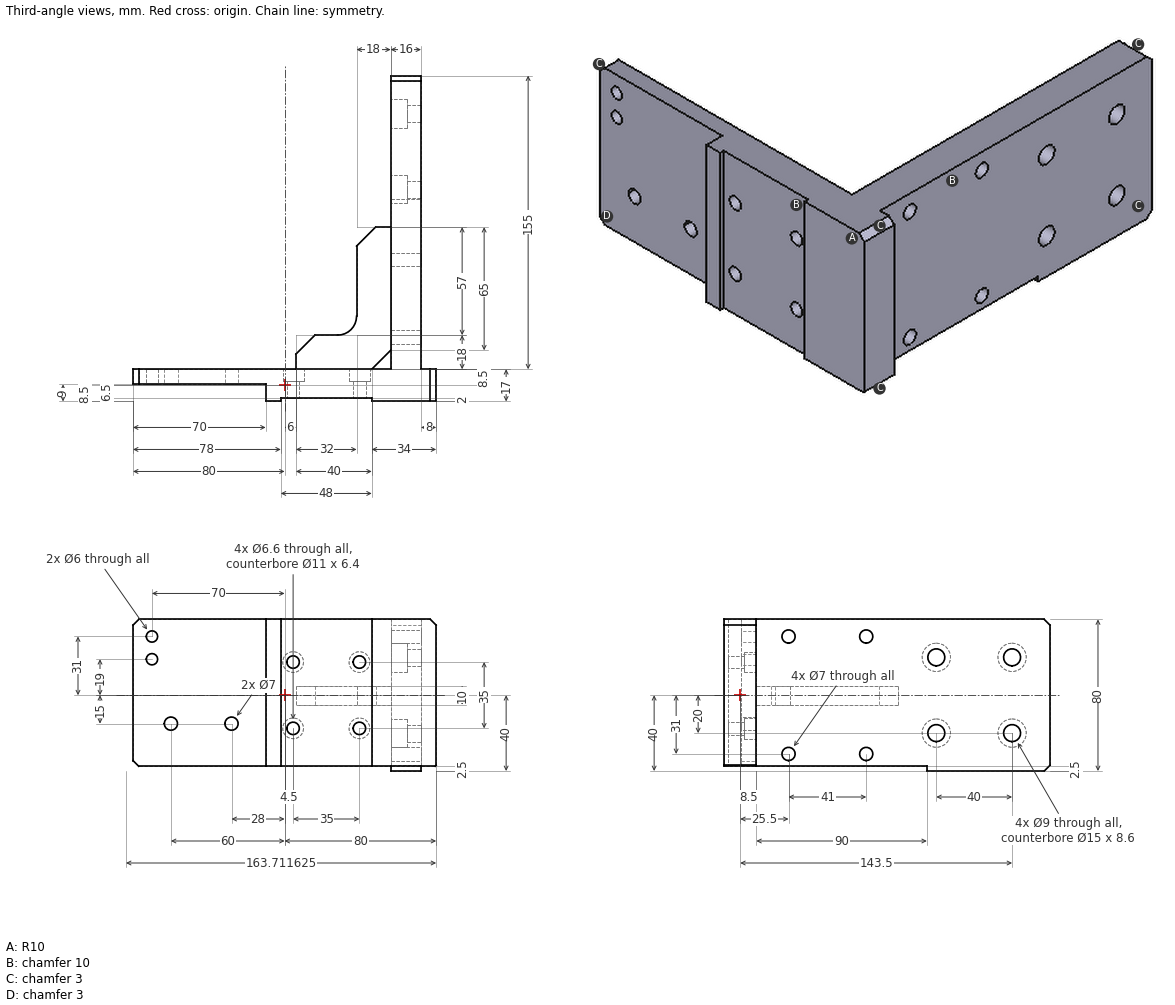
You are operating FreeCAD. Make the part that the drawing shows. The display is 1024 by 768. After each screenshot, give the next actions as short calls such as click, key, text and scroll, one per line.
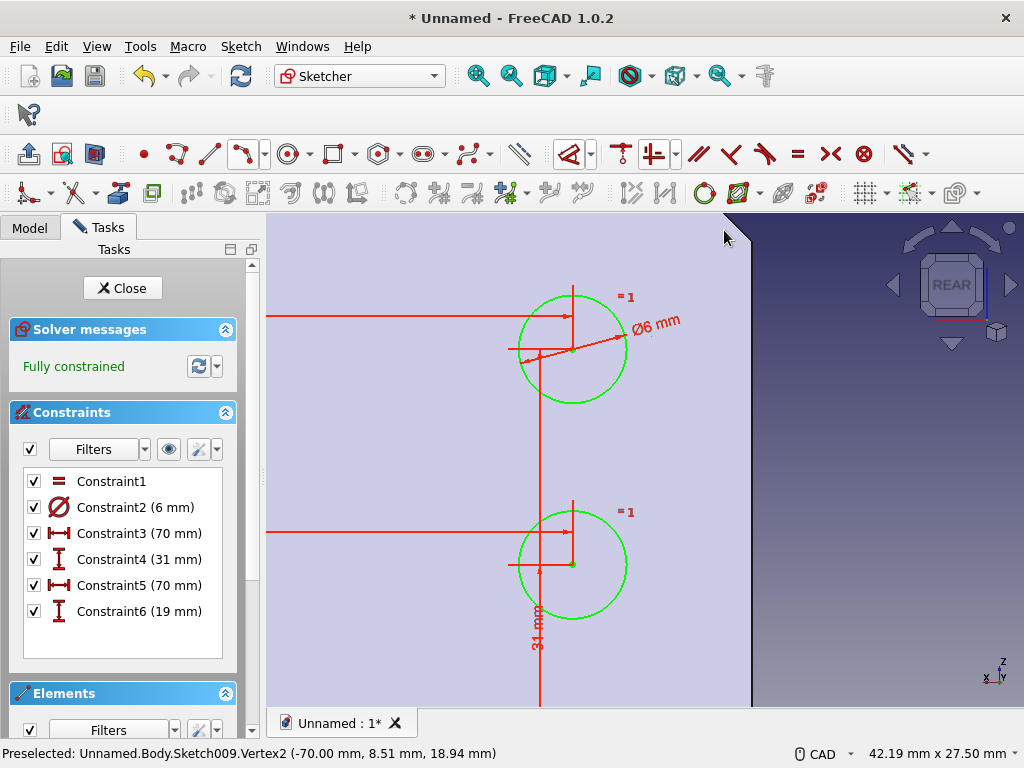
click(123, 288)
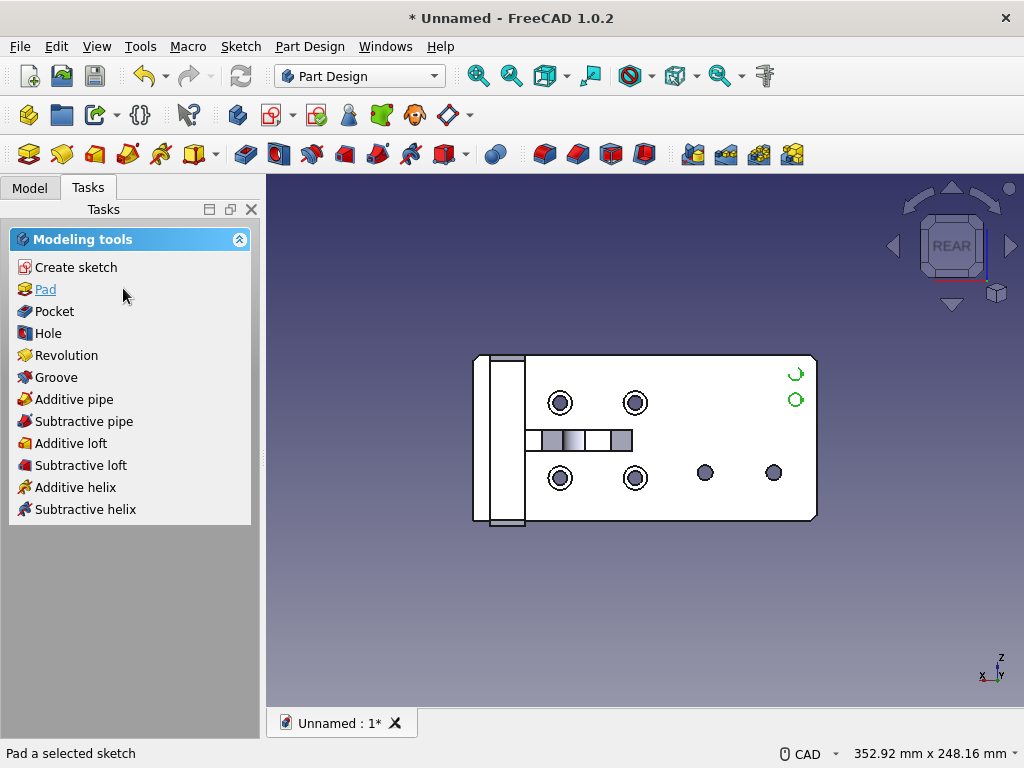
click(279, 154)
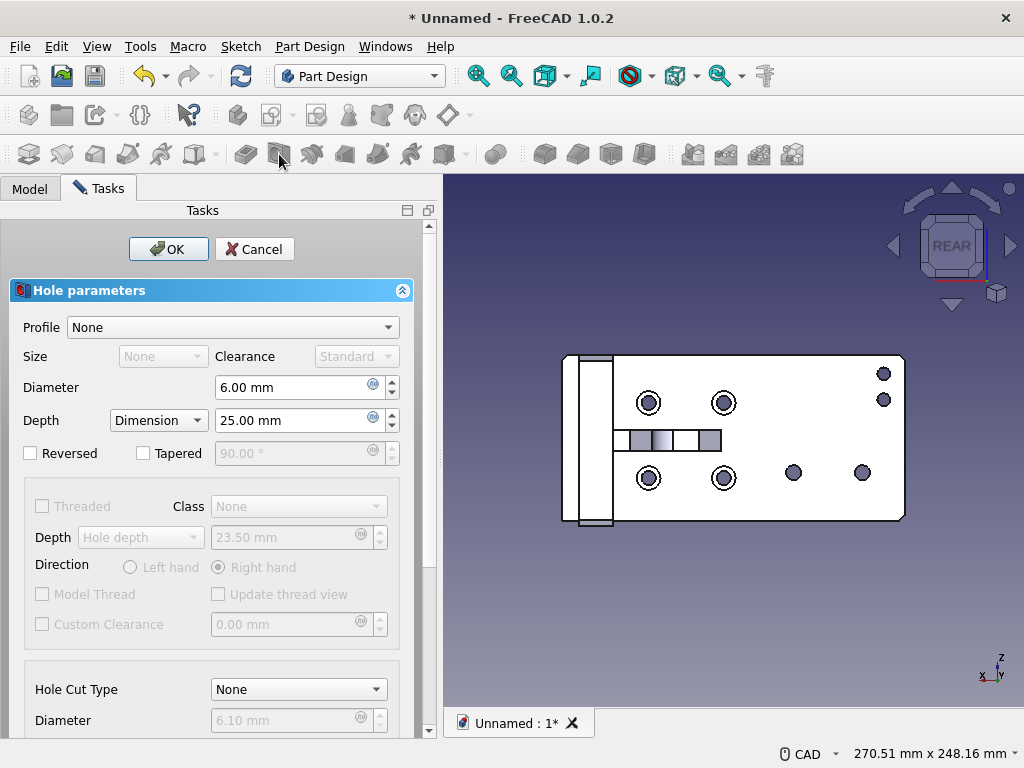
triple_click(300, 388)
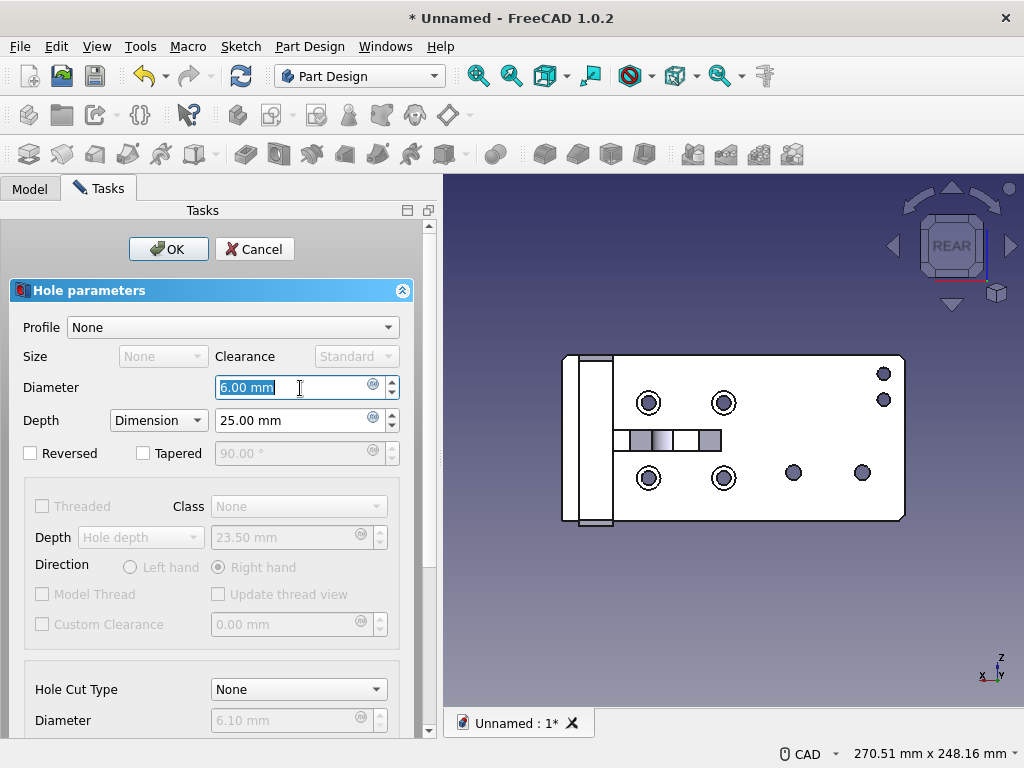
text(6)
key(Tab)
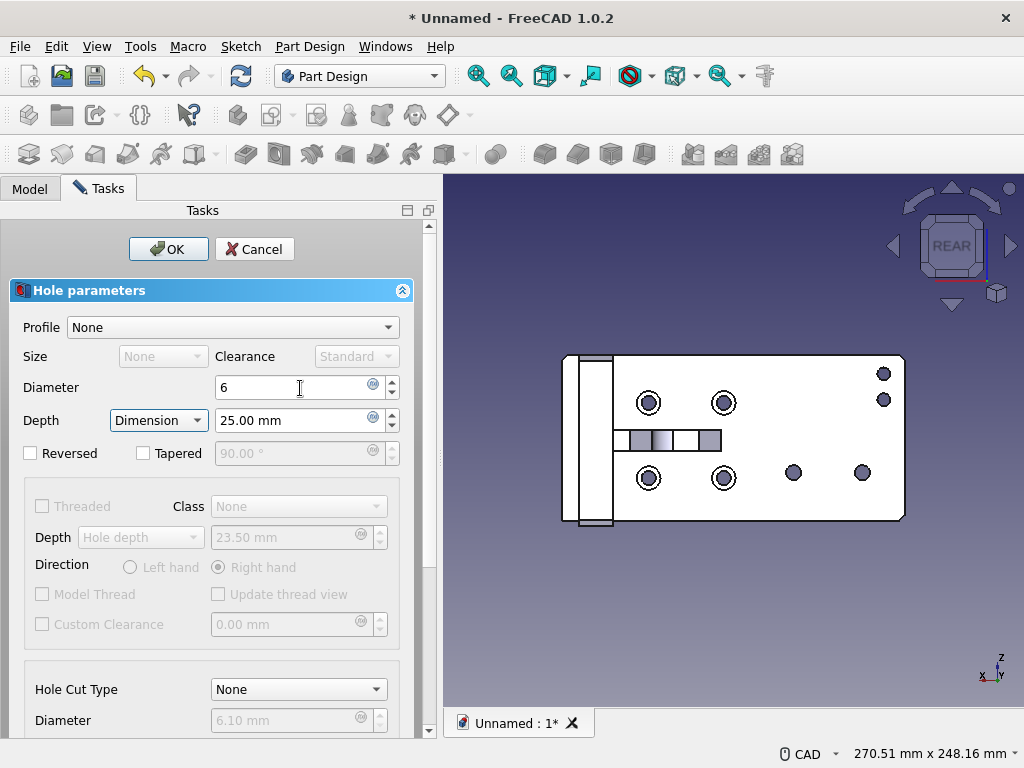
click(160, 420)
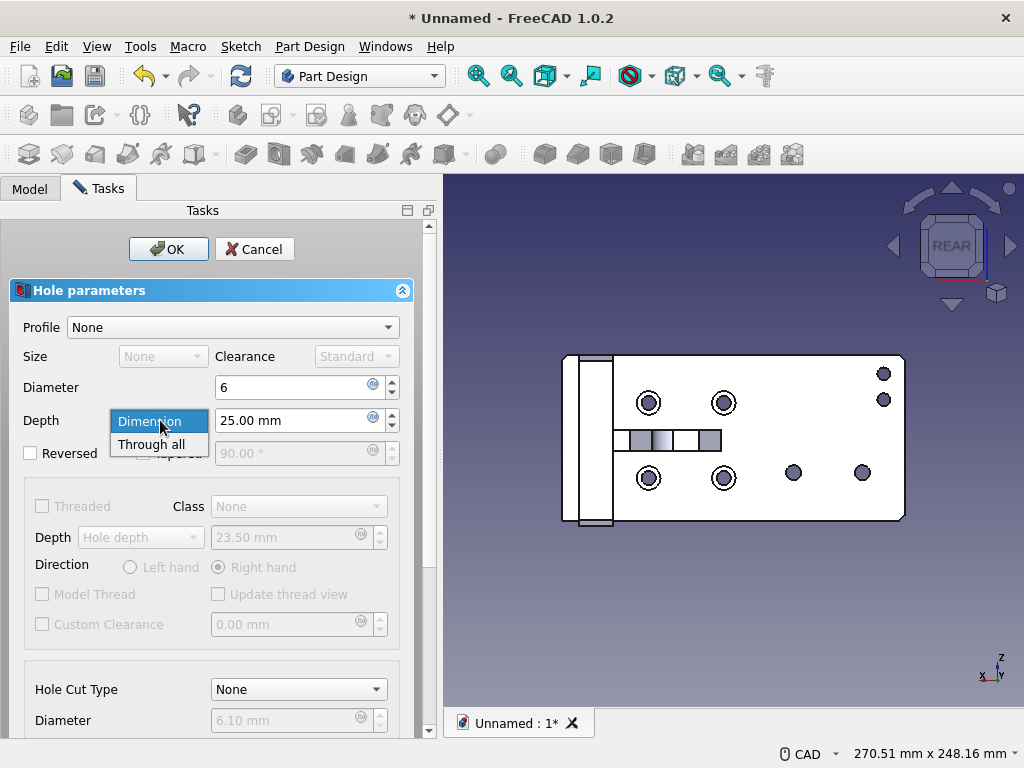
click(158, 444)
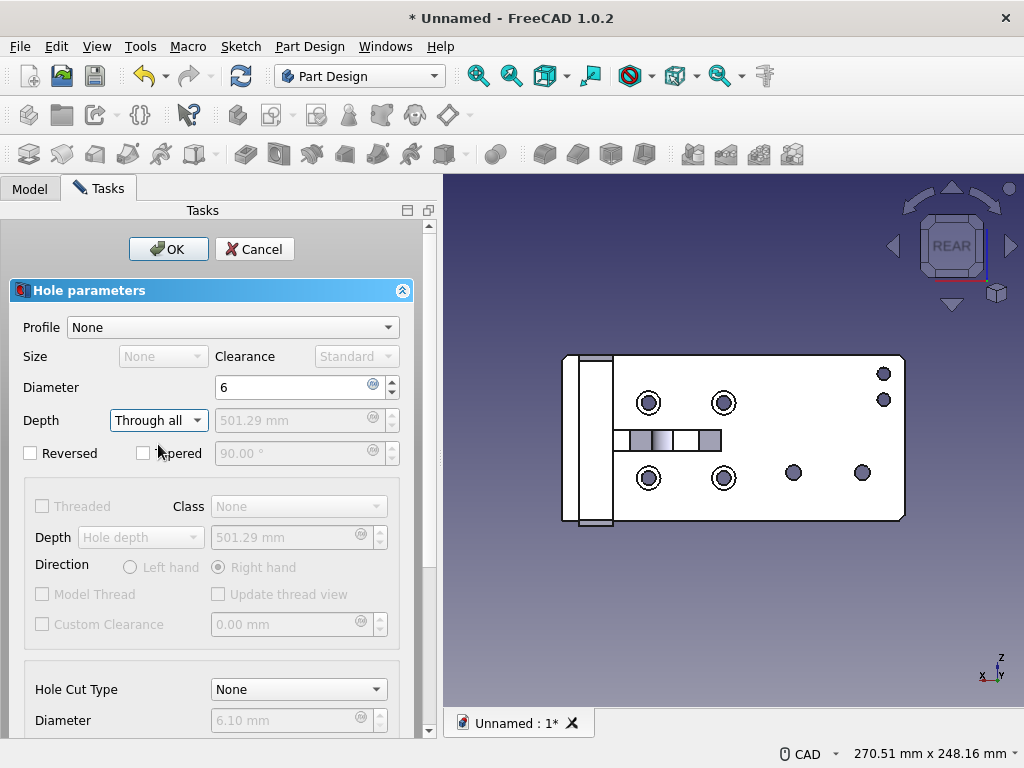
click(169, 249)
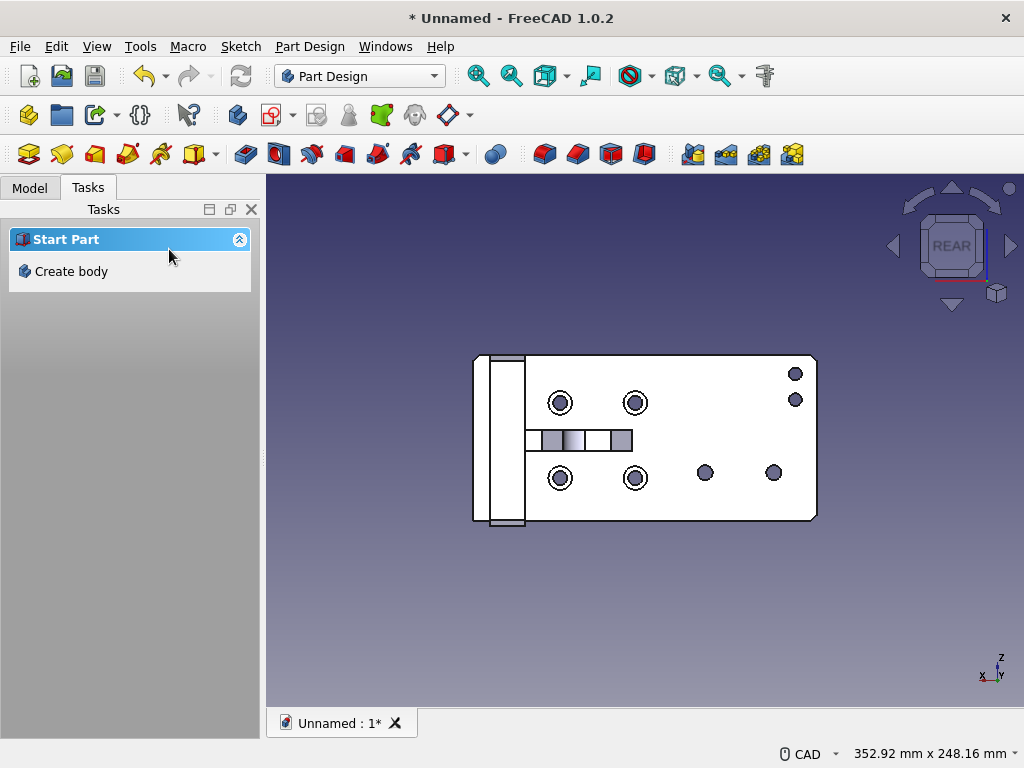
key(0)